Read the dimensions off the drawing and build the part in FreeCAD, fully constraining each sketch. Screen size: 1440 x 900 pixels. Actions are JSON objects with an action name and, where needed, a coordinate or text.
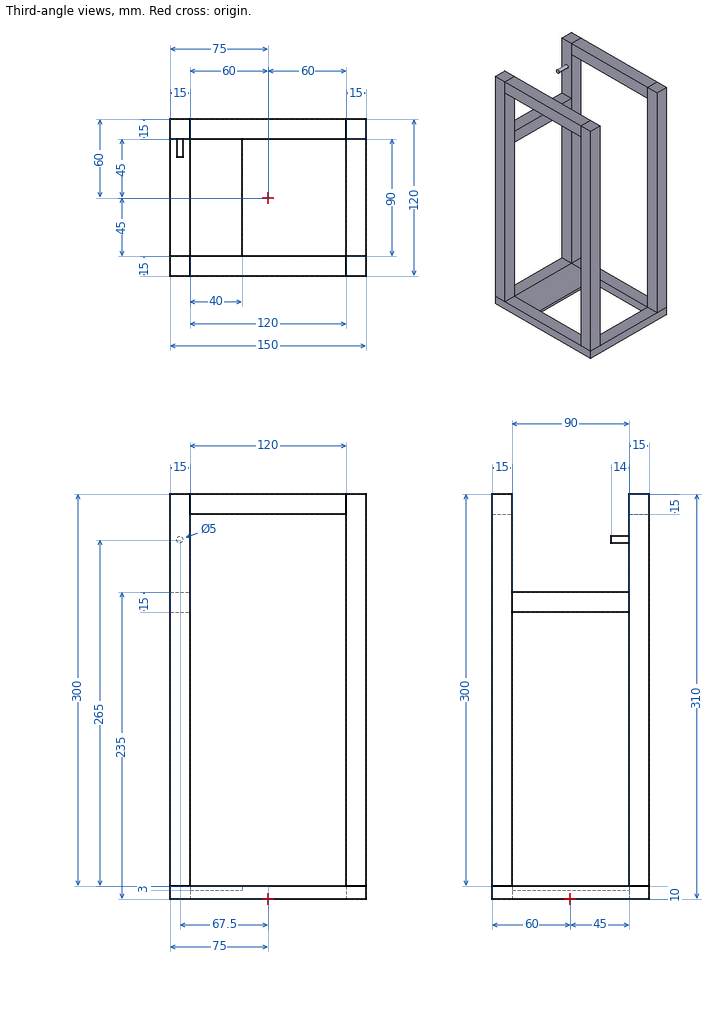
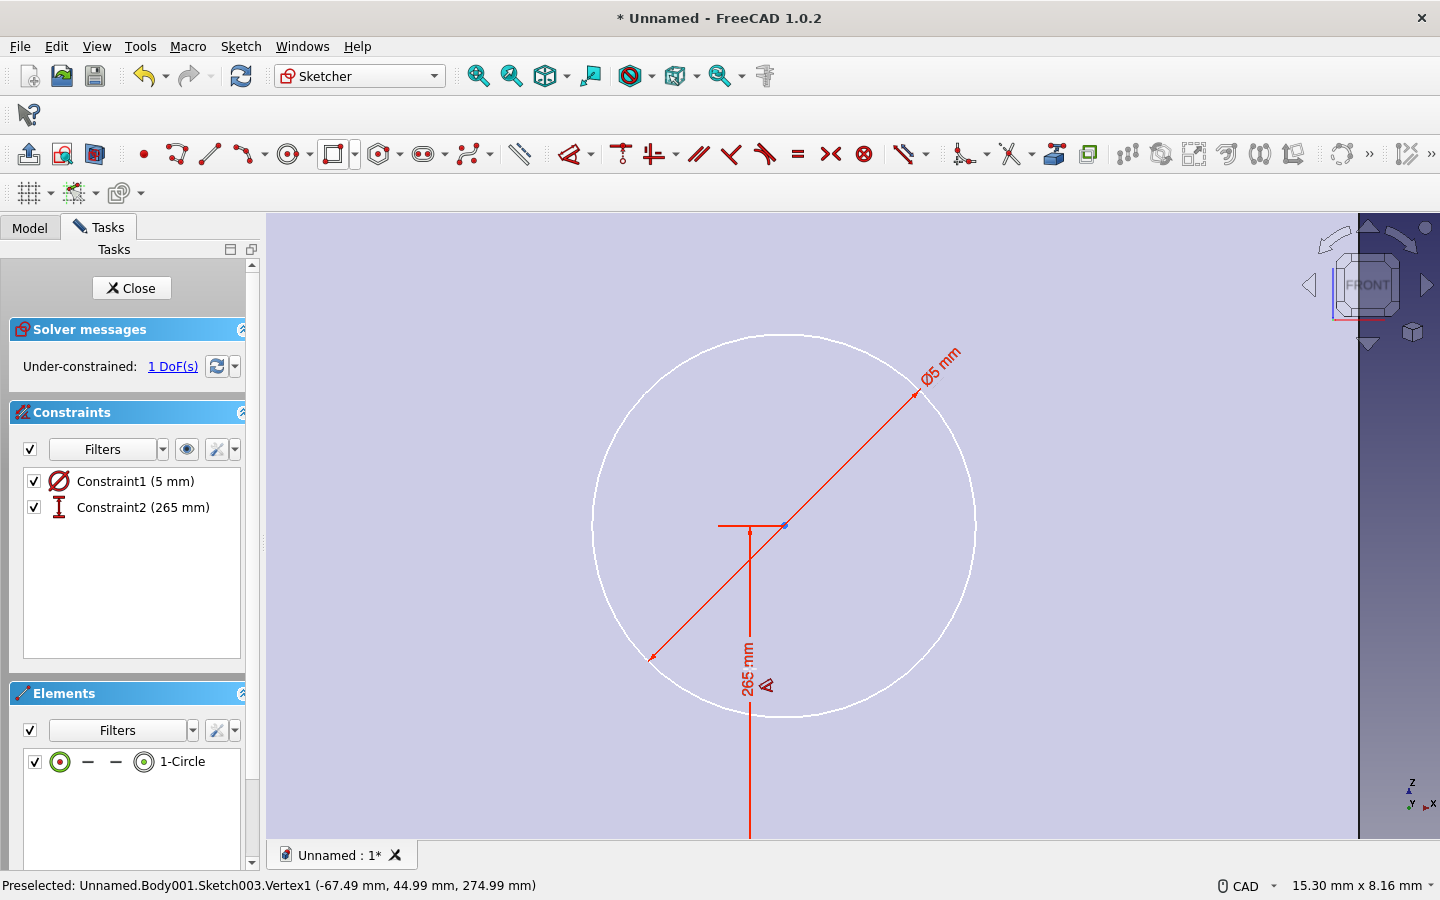
{"action": "left_click", "coordinate": [784, 526]}
{"action": "left_click", "coordinate": [1029, 492]}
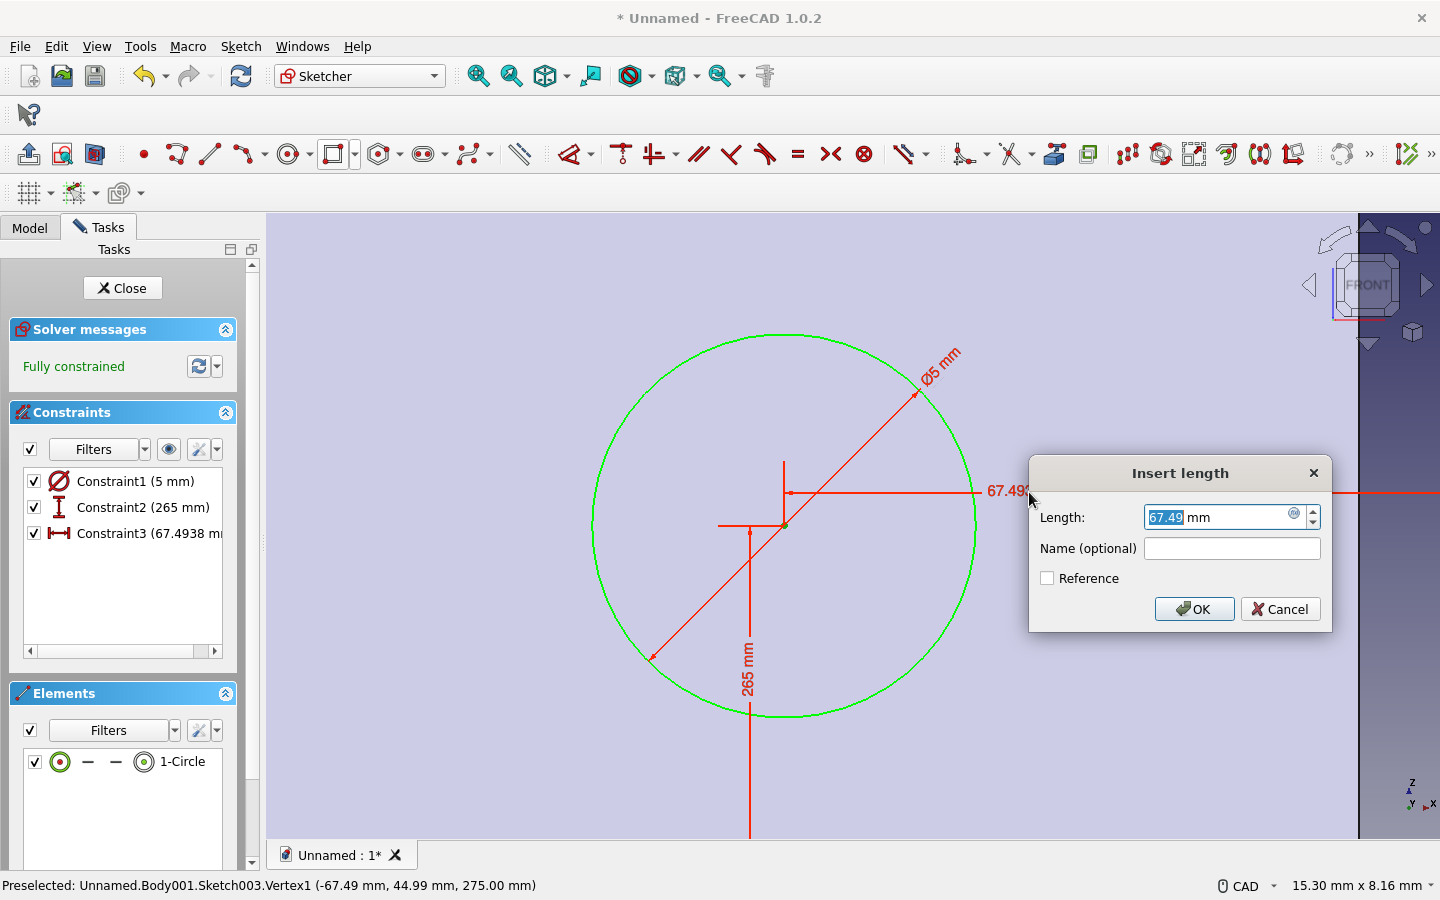
{"action": "type", "text": "67.5"}
{"action": "key", "text": "Return"}
{"action": "key", "text": "Escape"}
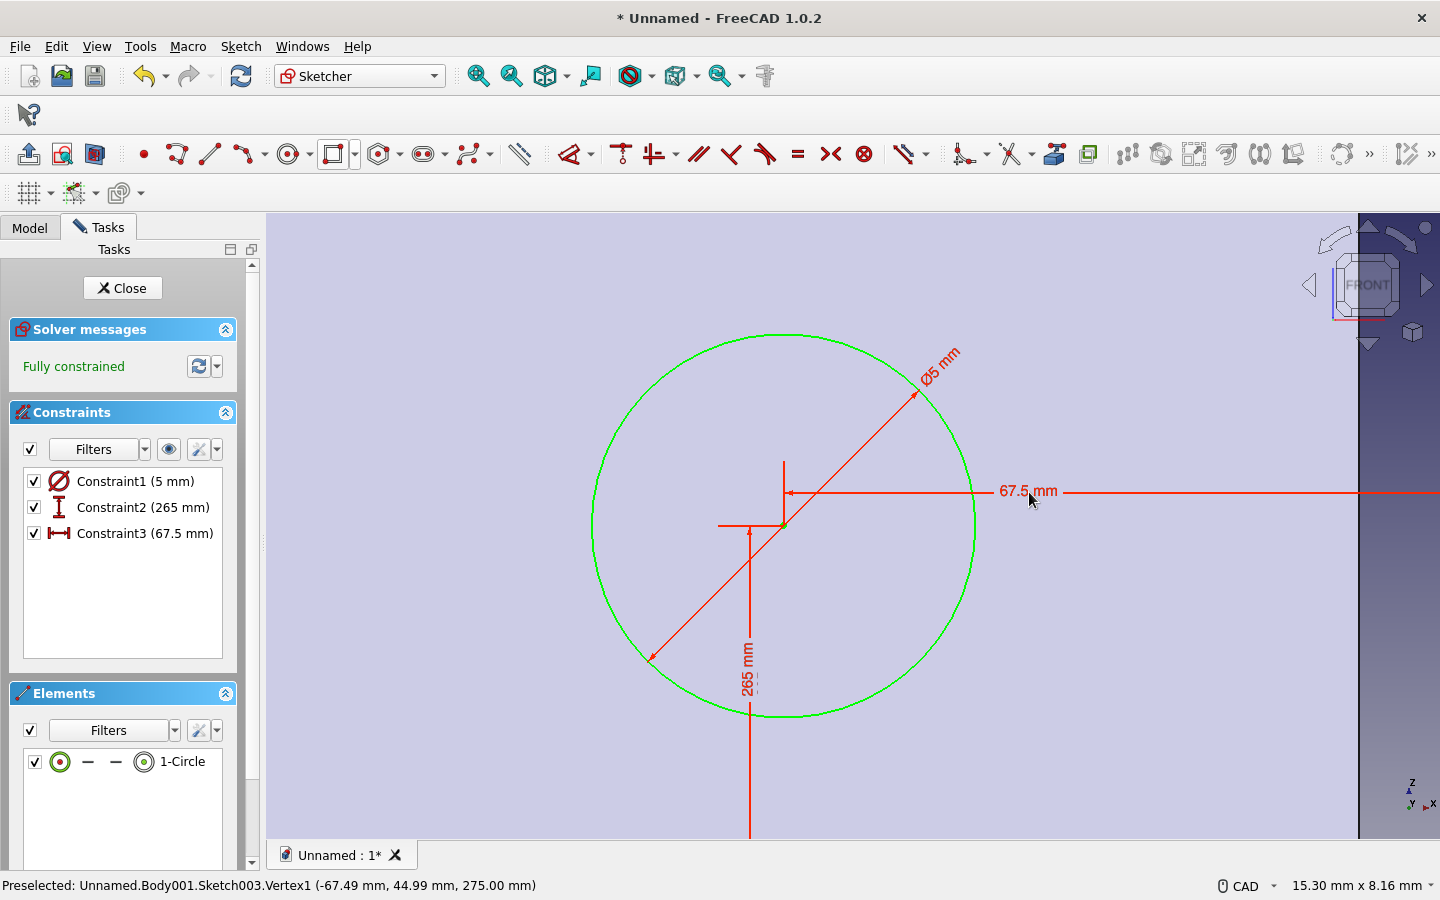
{"action": "left_click", "coordinate": [123, 288]}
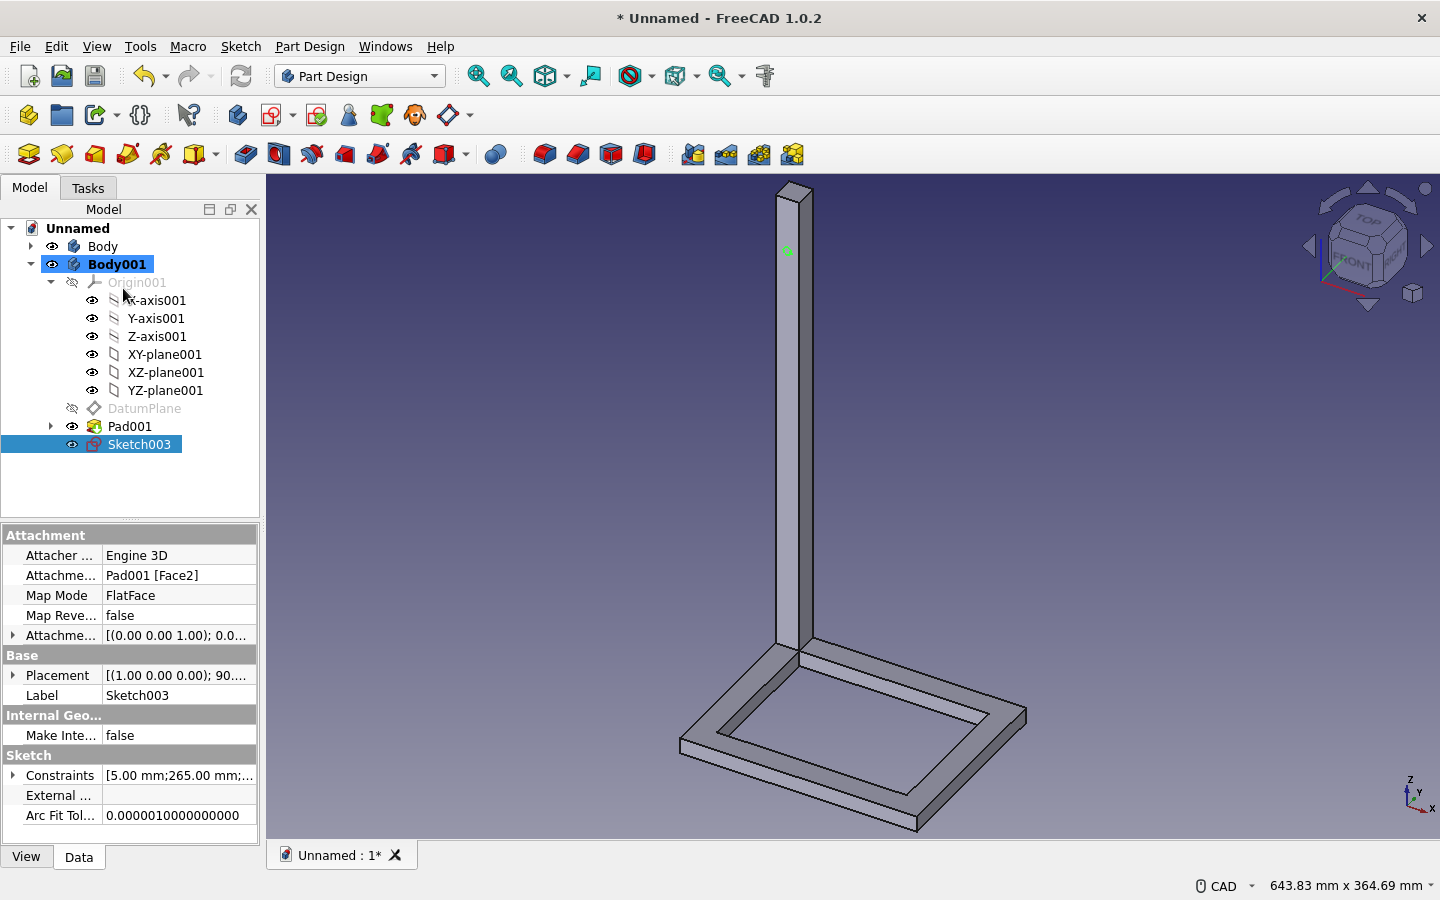
{"action": "left_click", "coordinate": [29, 154]}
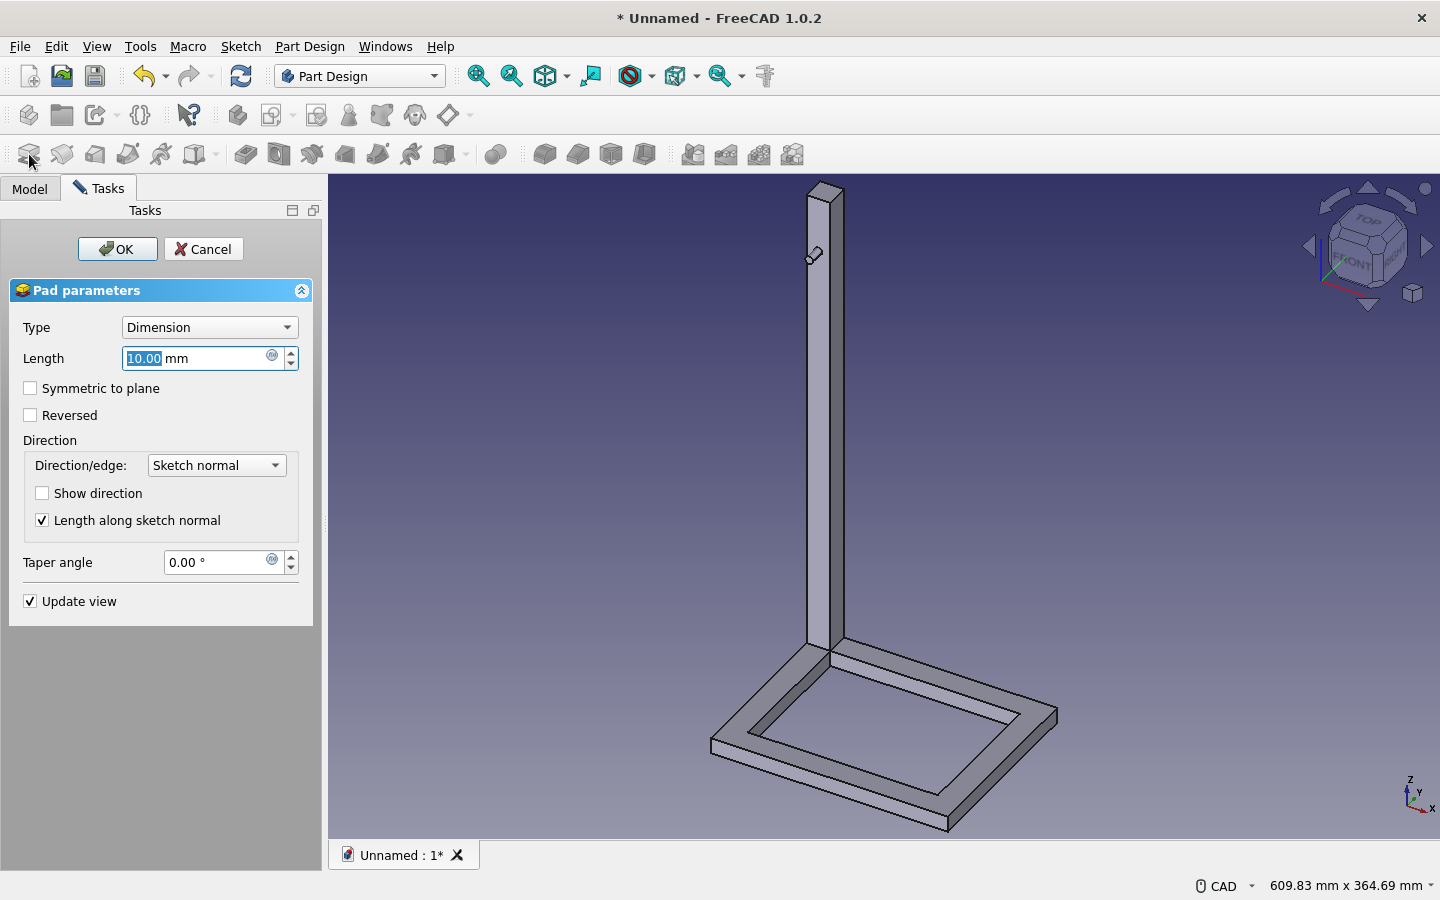
{"action": "type", "text": "14"}
{"action": "key", "text": "Tab"}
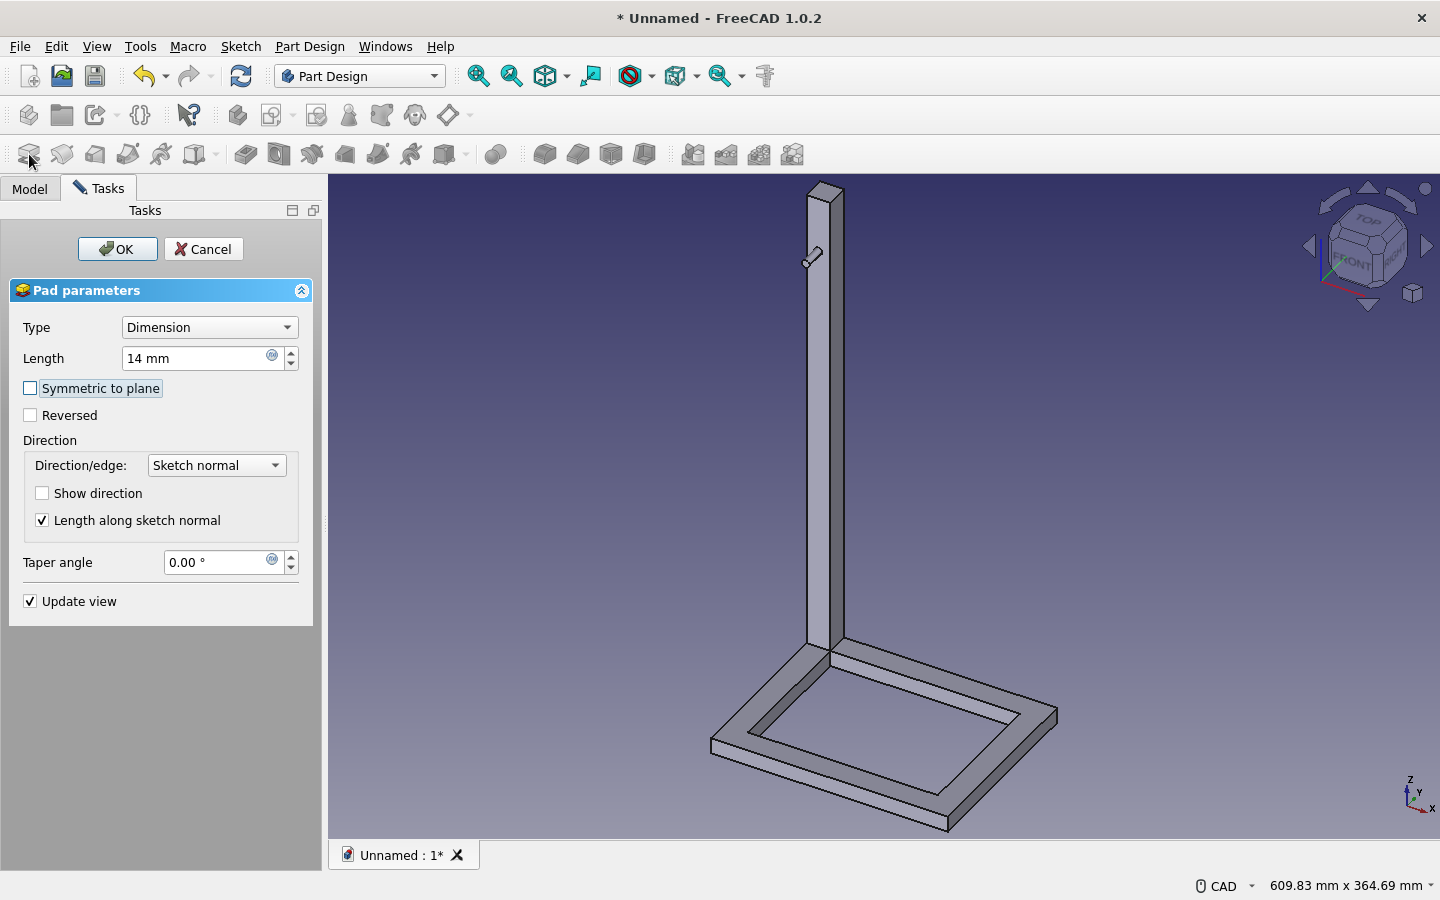
{"action": "left_click", "coordinate": [118, 249]}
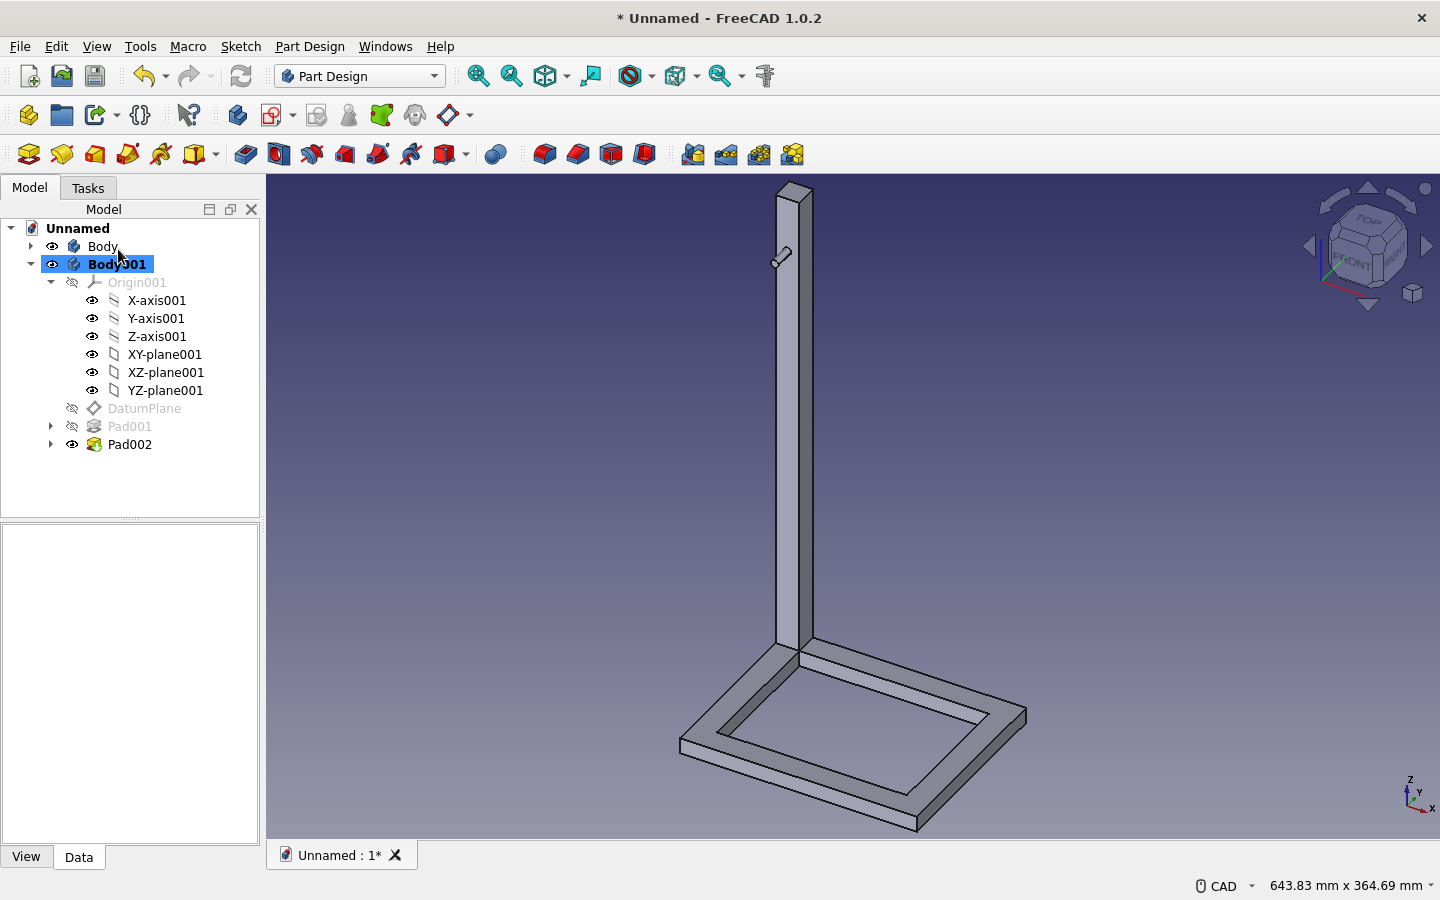
{"action": "left_click", "coordinate": [238, 116]}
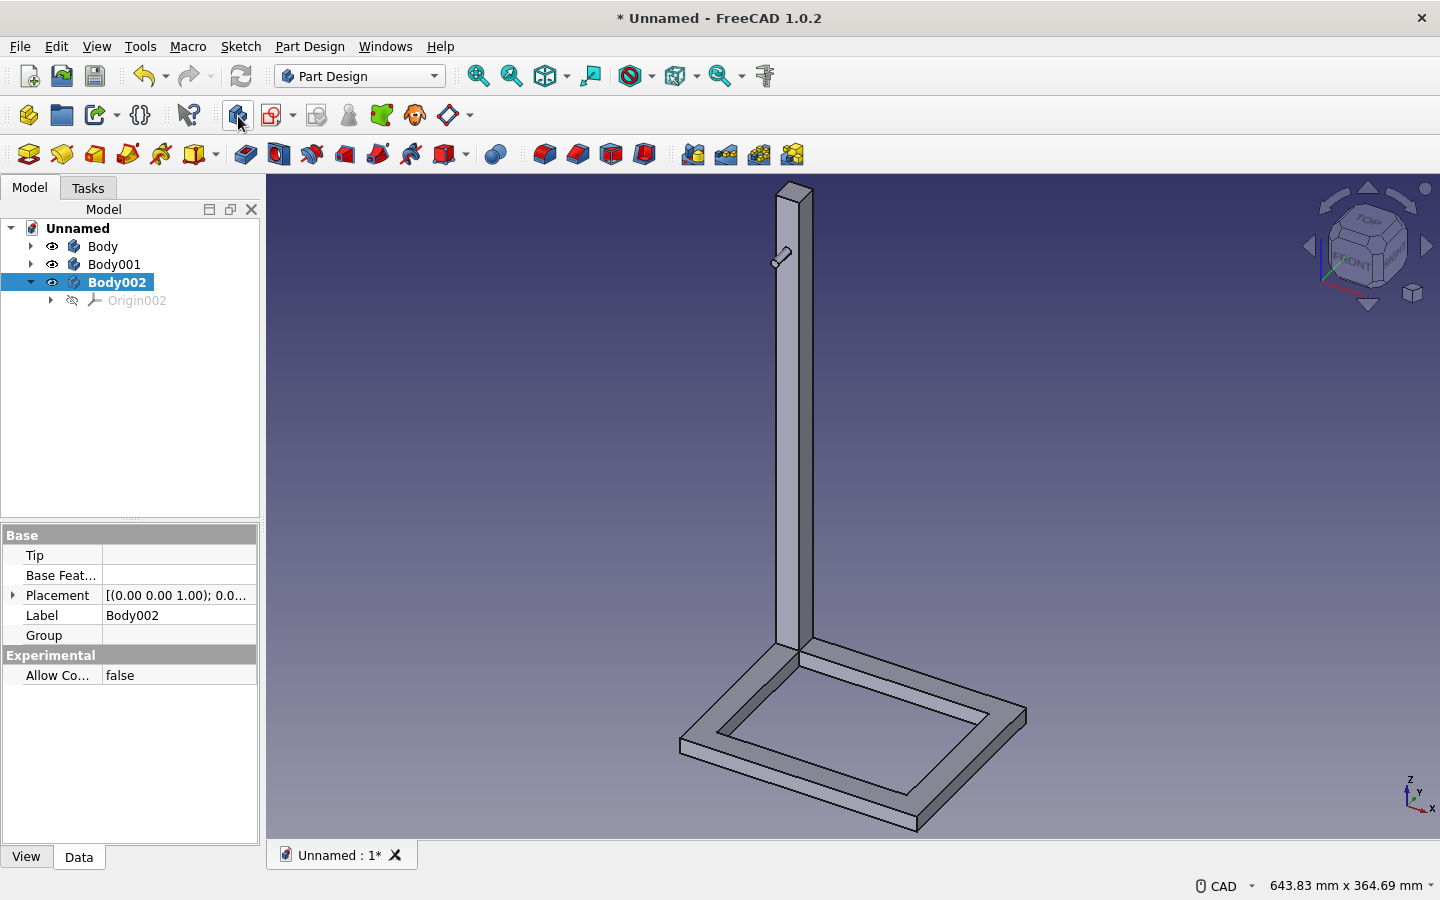
{"action": "left_click", "coordinate": [51, 300]}